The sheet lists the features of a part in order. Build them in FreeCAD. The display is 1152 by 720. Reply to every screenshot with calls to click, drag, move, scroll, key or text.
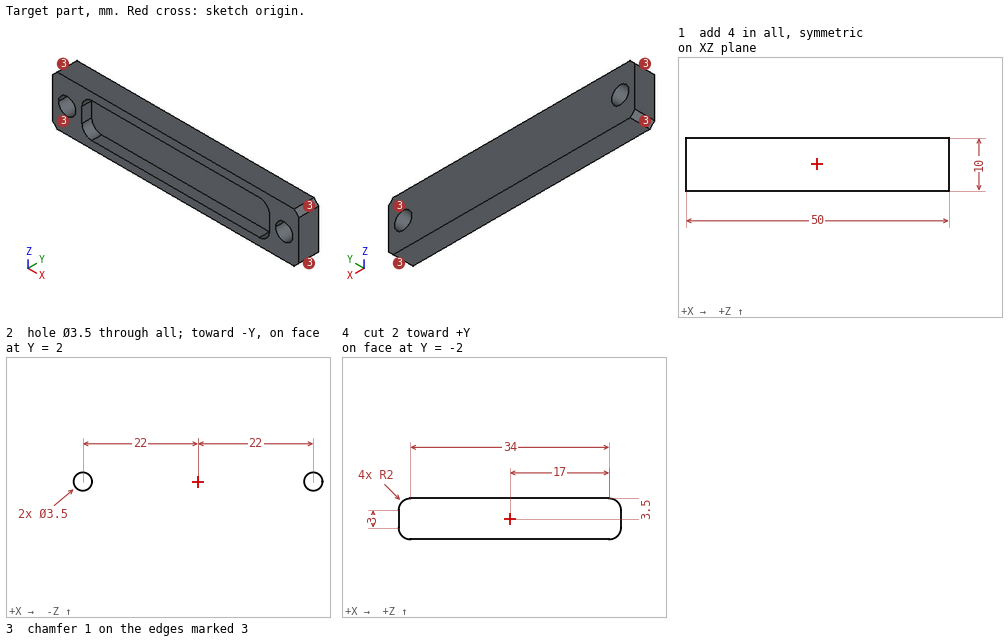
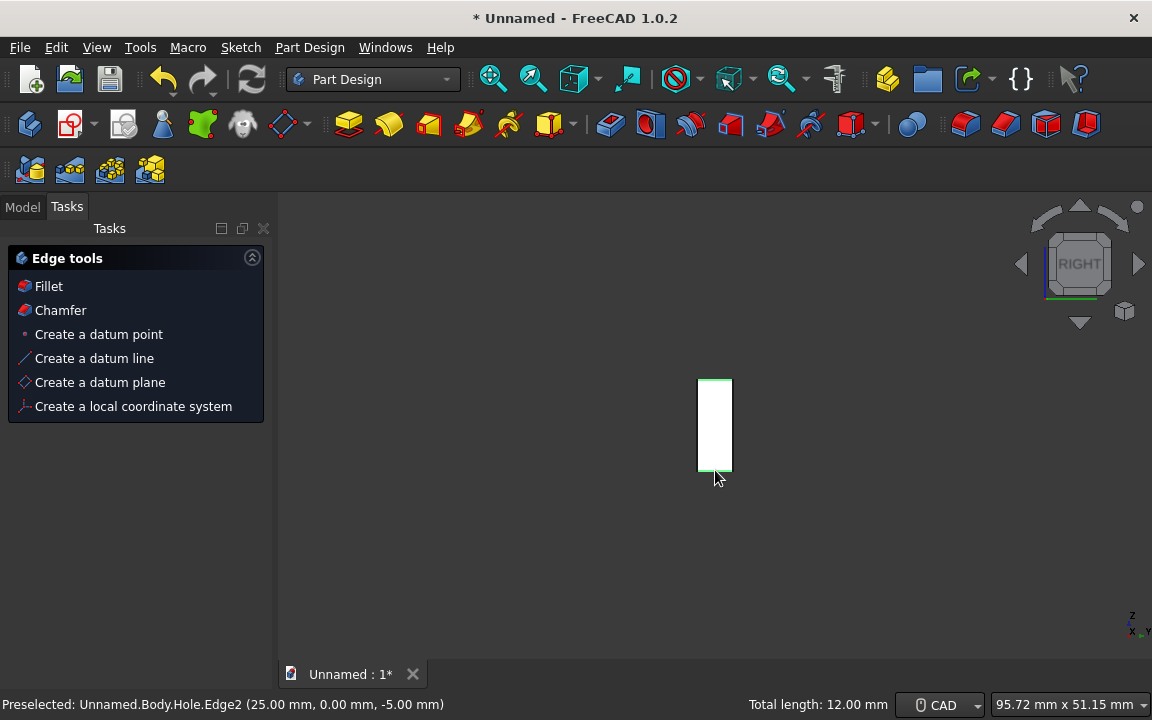
key(5)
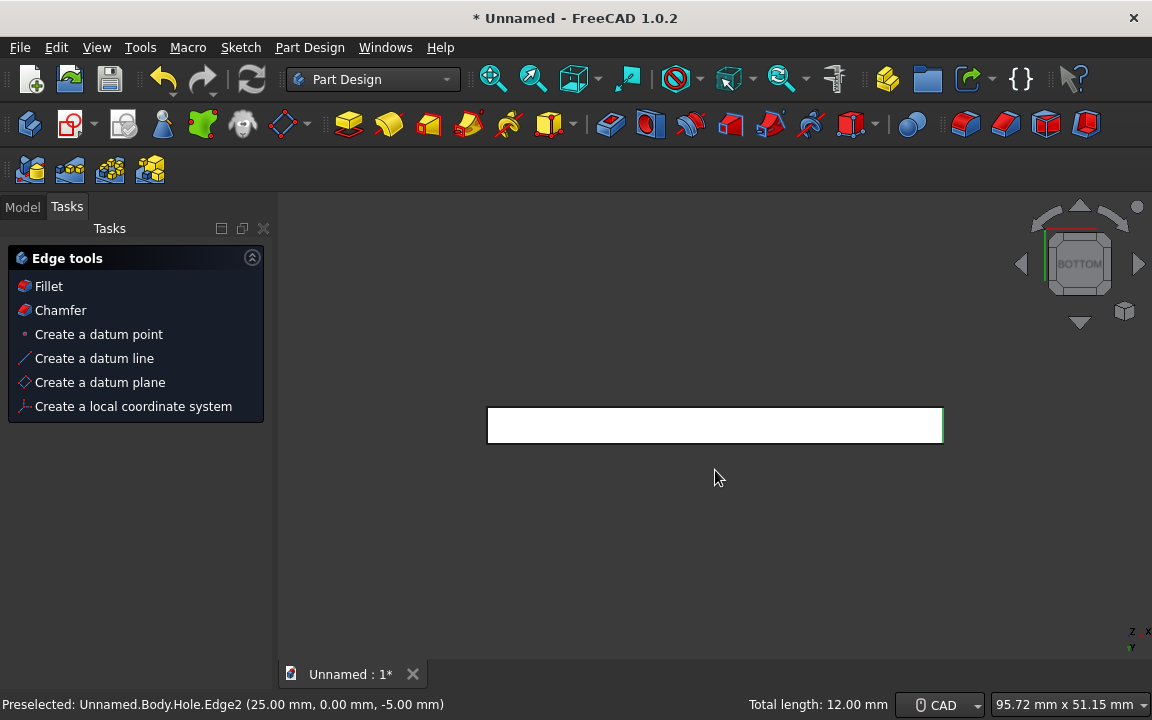
click(487, 424, ctrl)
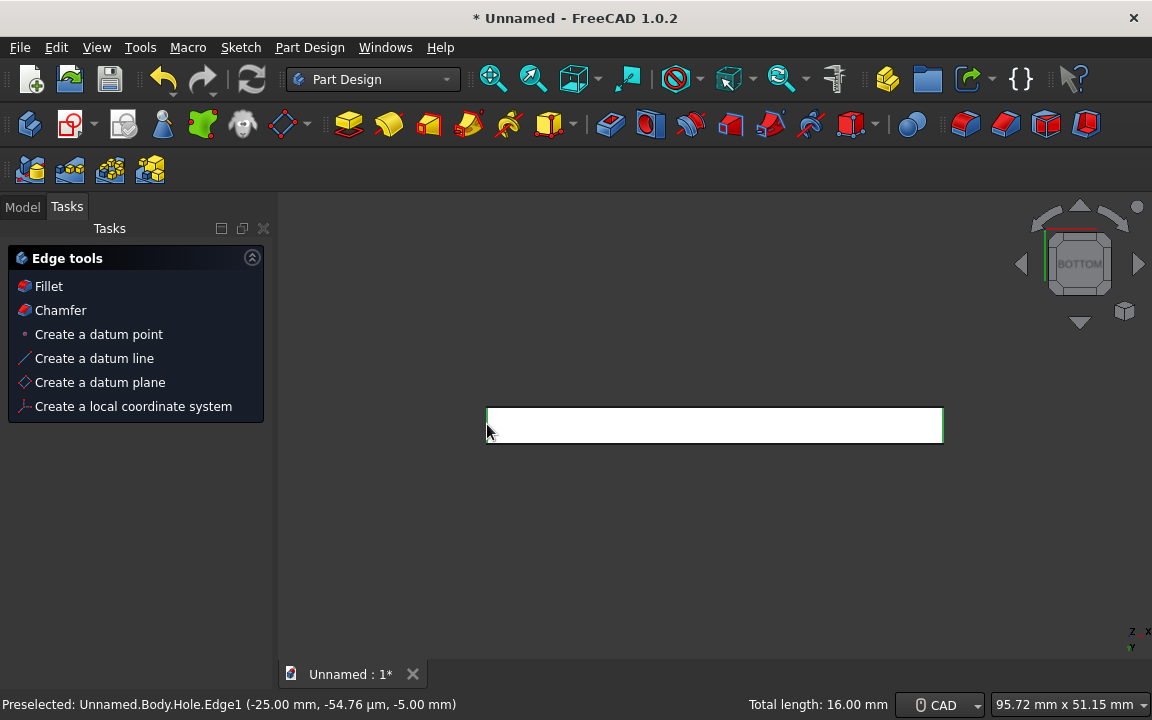
click(1006, 124)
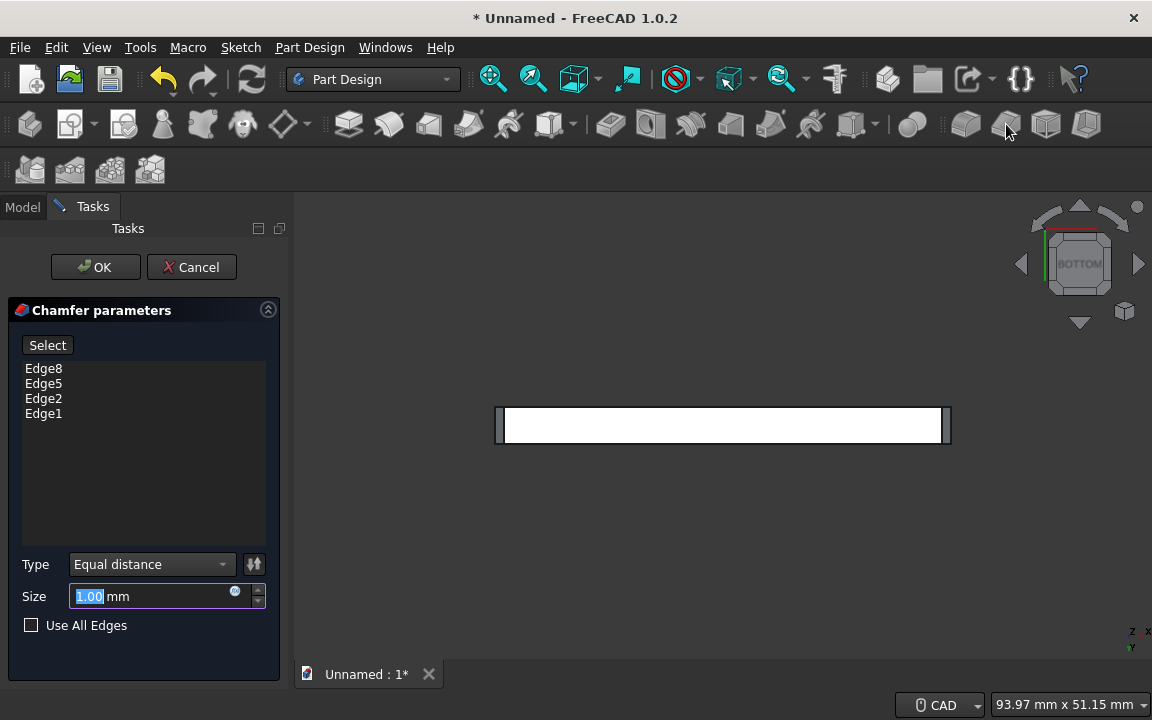
text(1)
key(Tab)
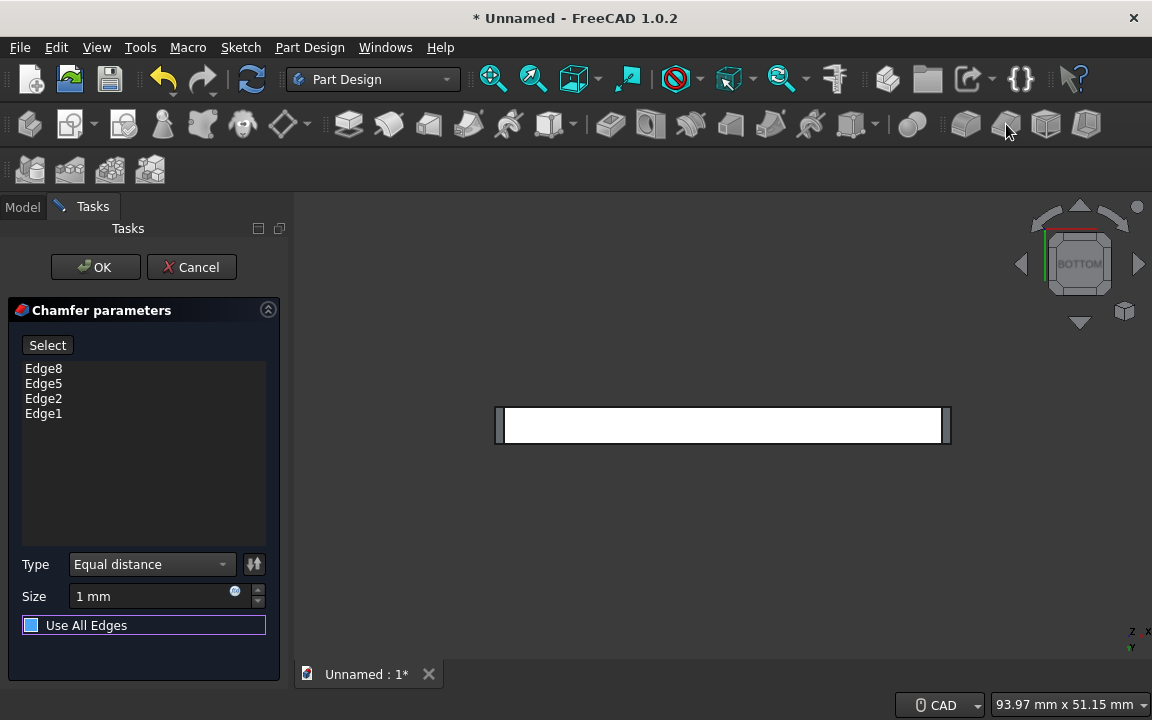
click(96, 267)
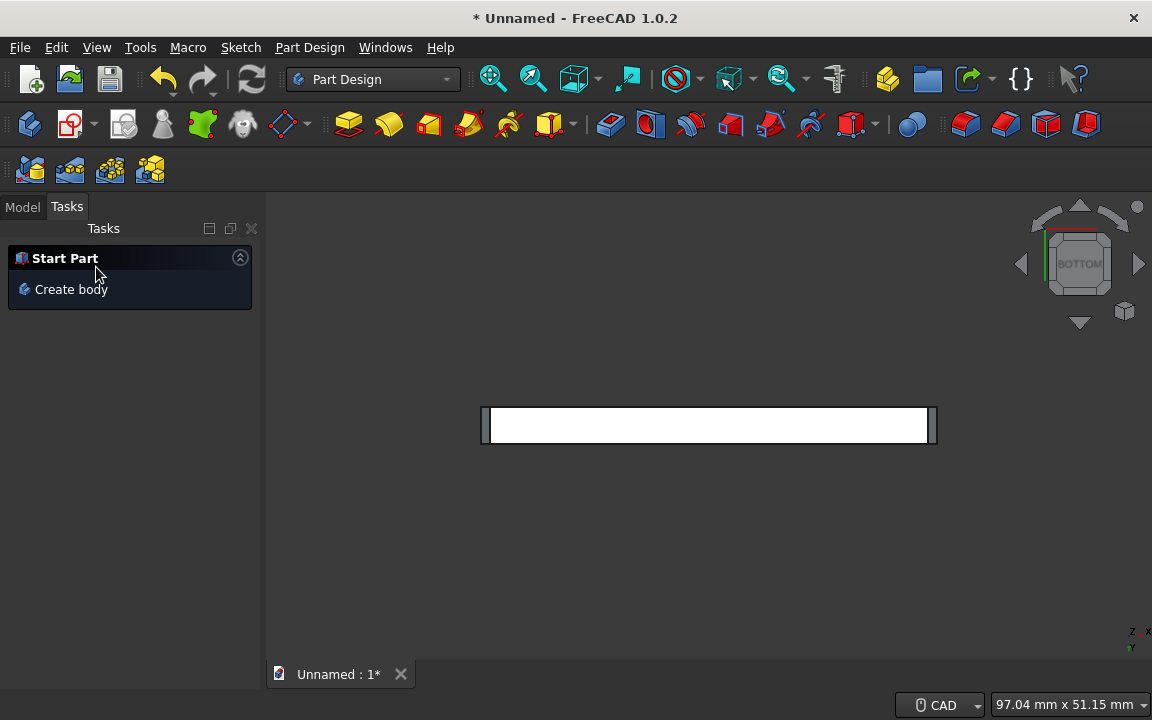
key(0)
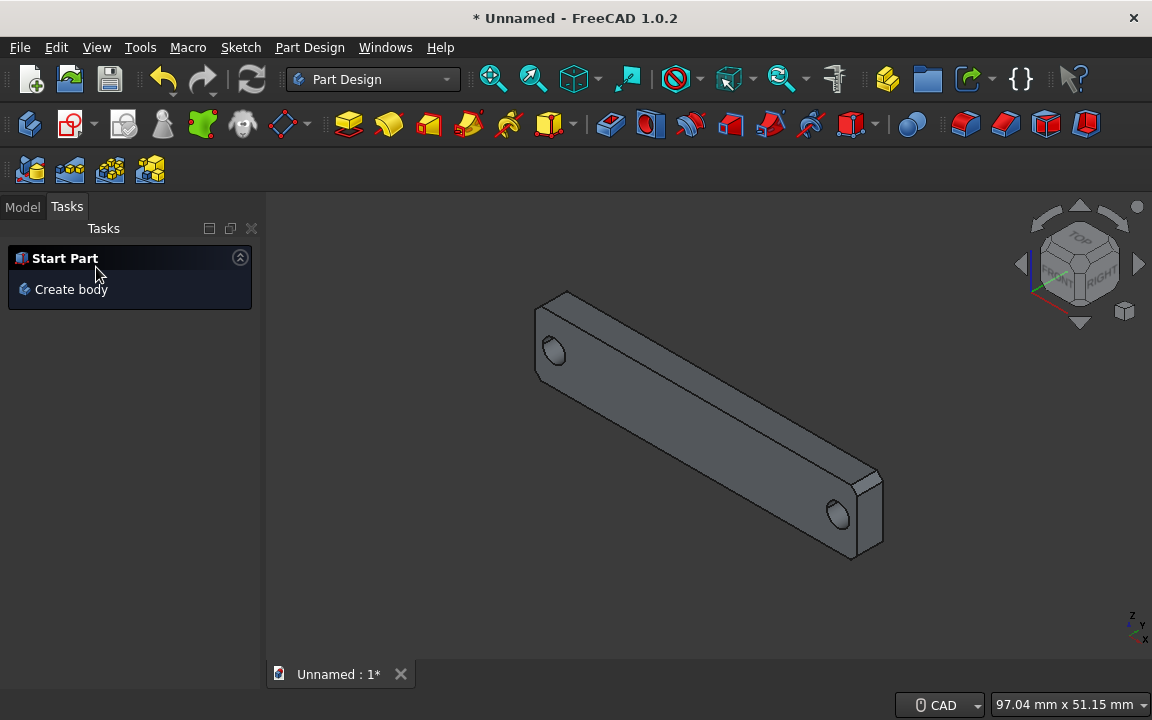
click(788, 485)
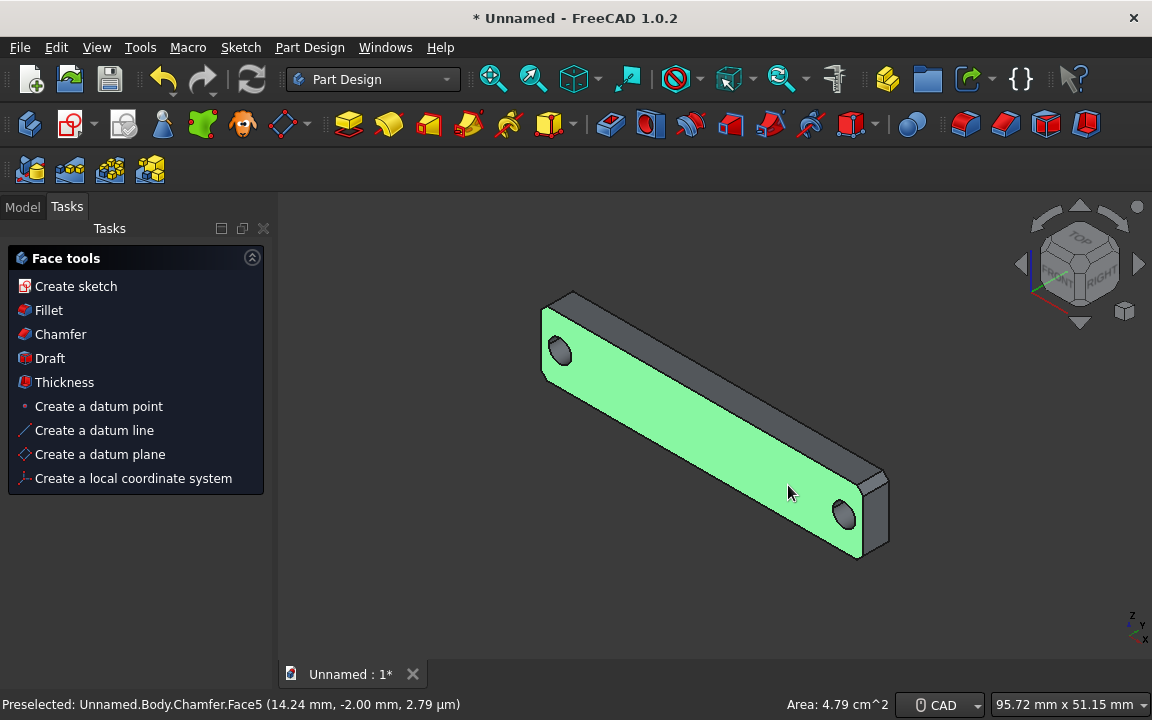
click(70, 124)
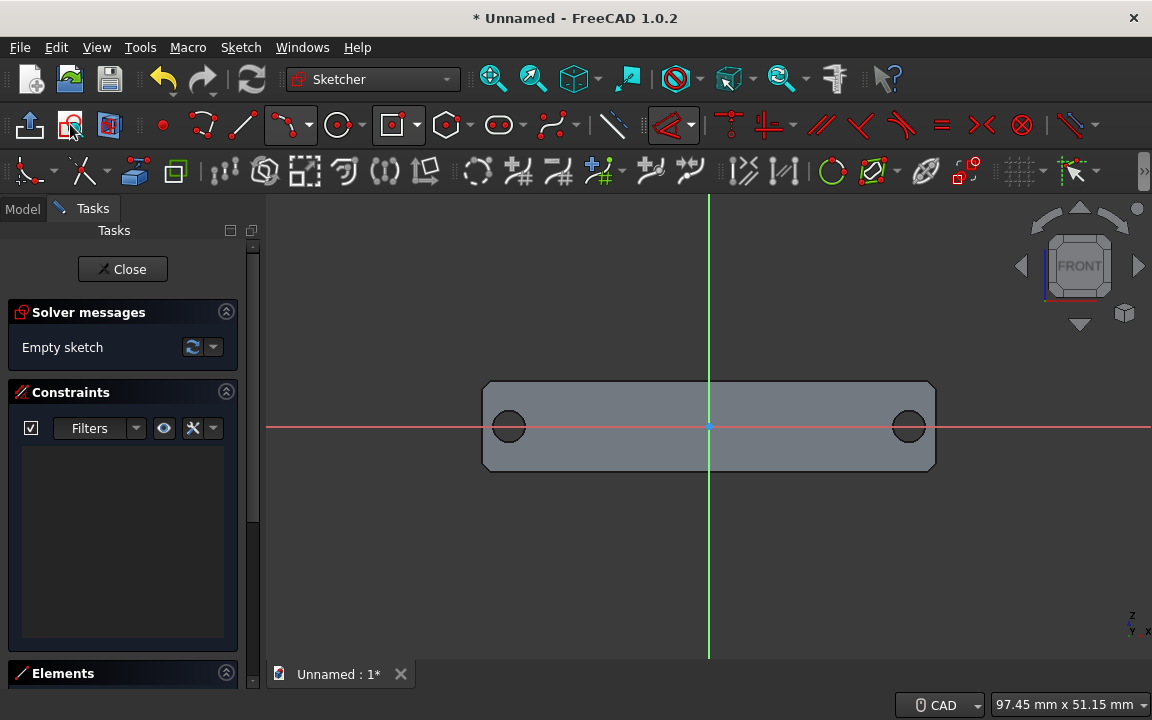
scroll(848, 426, up, 2)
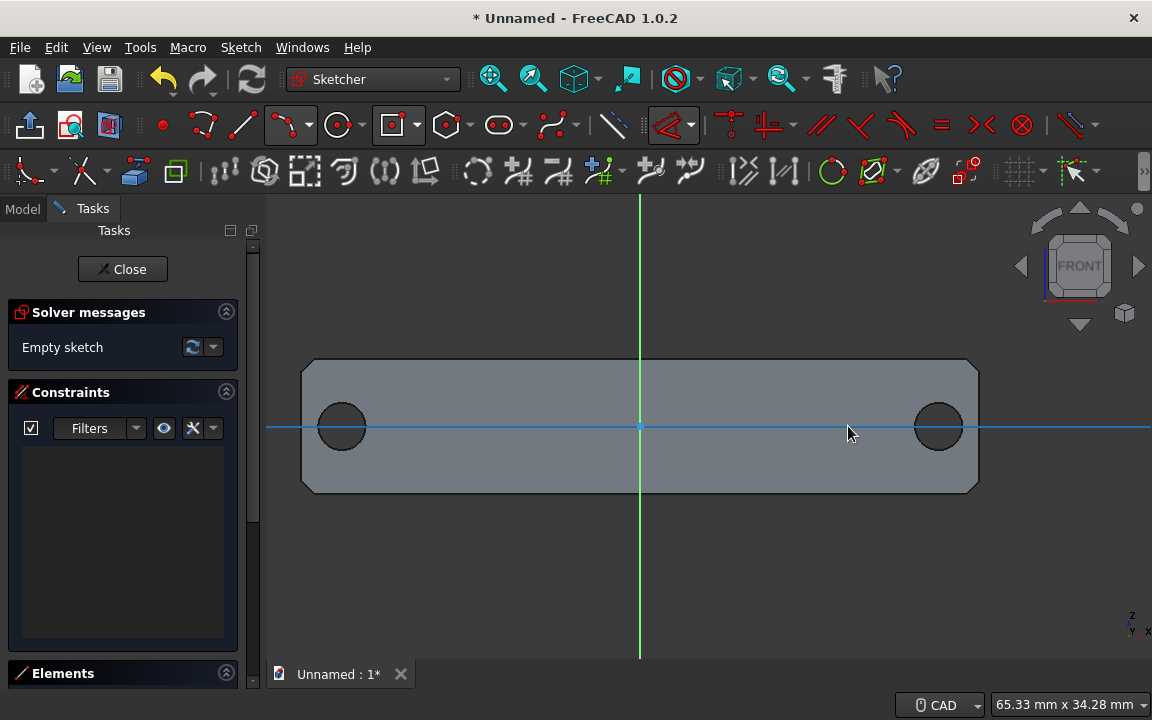
click(244, 126)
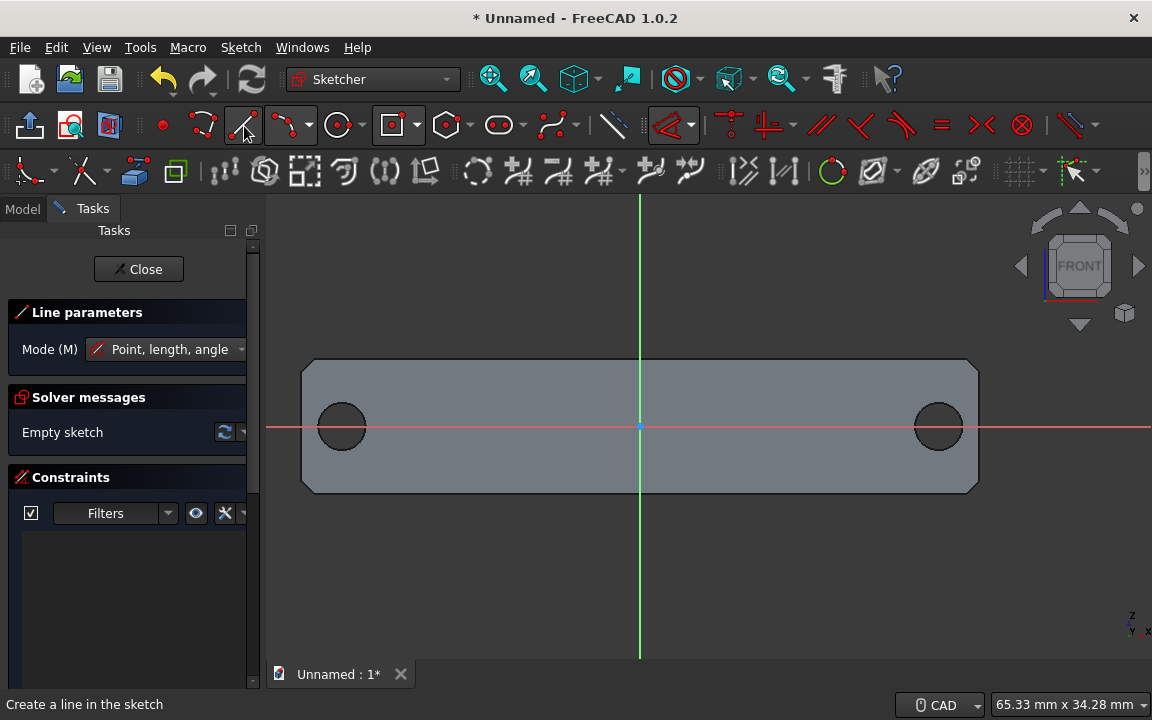
click(871, 379)
click(410, 379)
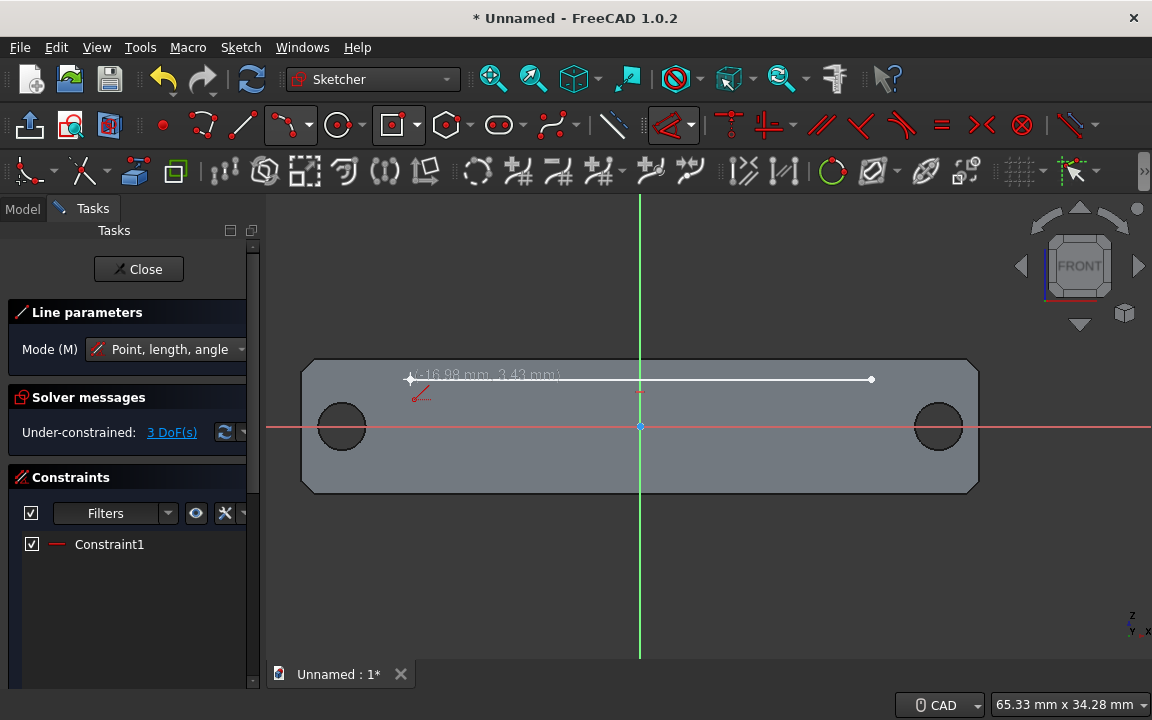
click(383, 406)
click(383, 447)